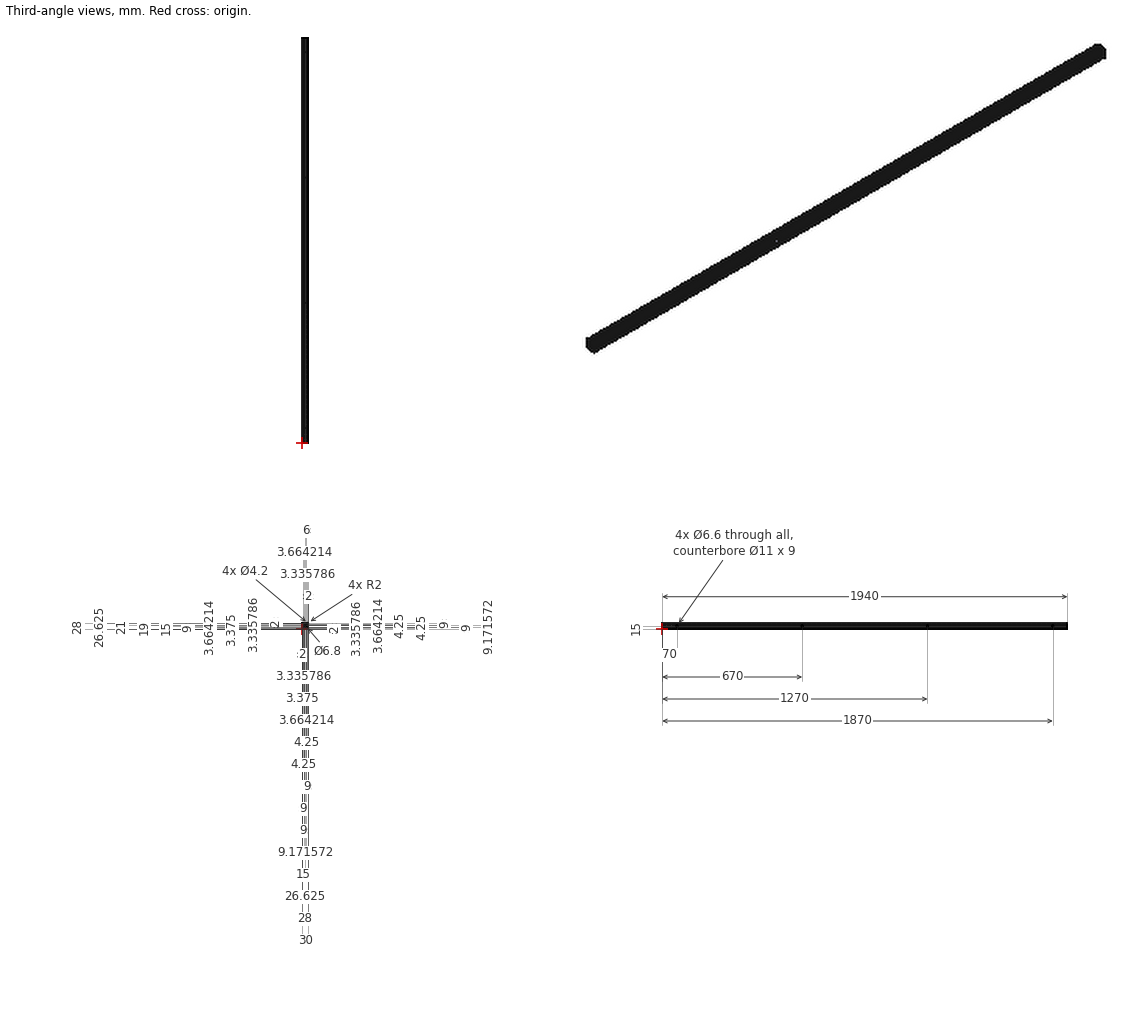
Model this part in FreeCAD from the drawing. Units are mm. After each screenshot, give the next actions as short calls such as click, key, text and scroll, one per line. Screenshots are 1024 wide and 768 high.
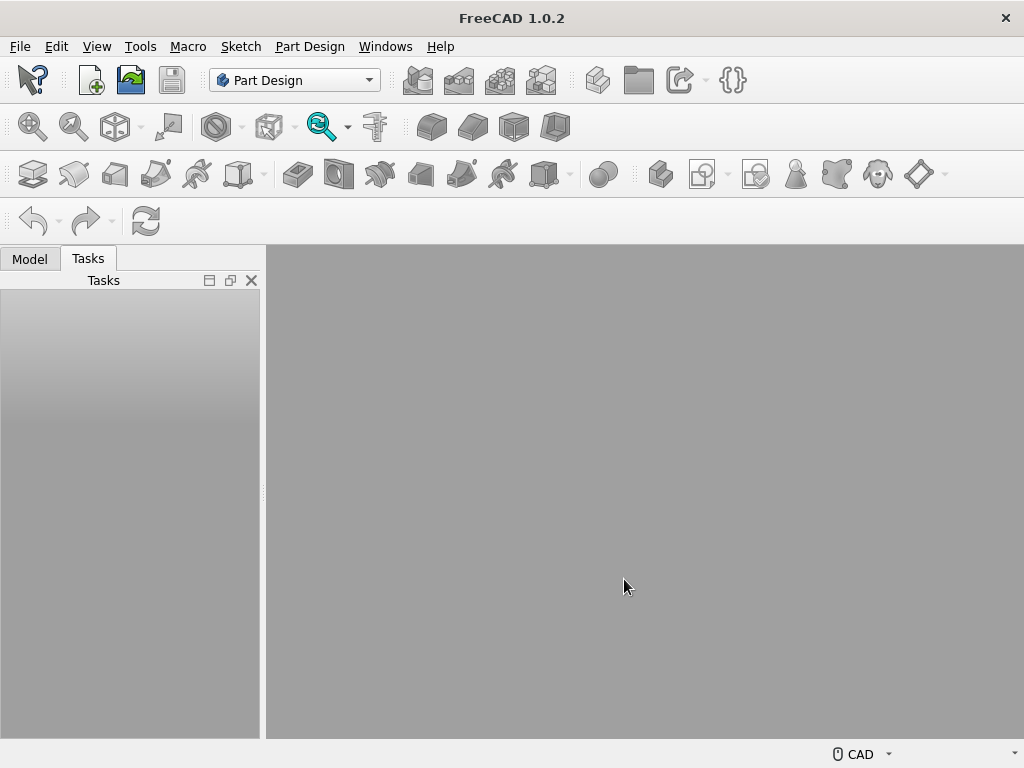
key(ctrl+n)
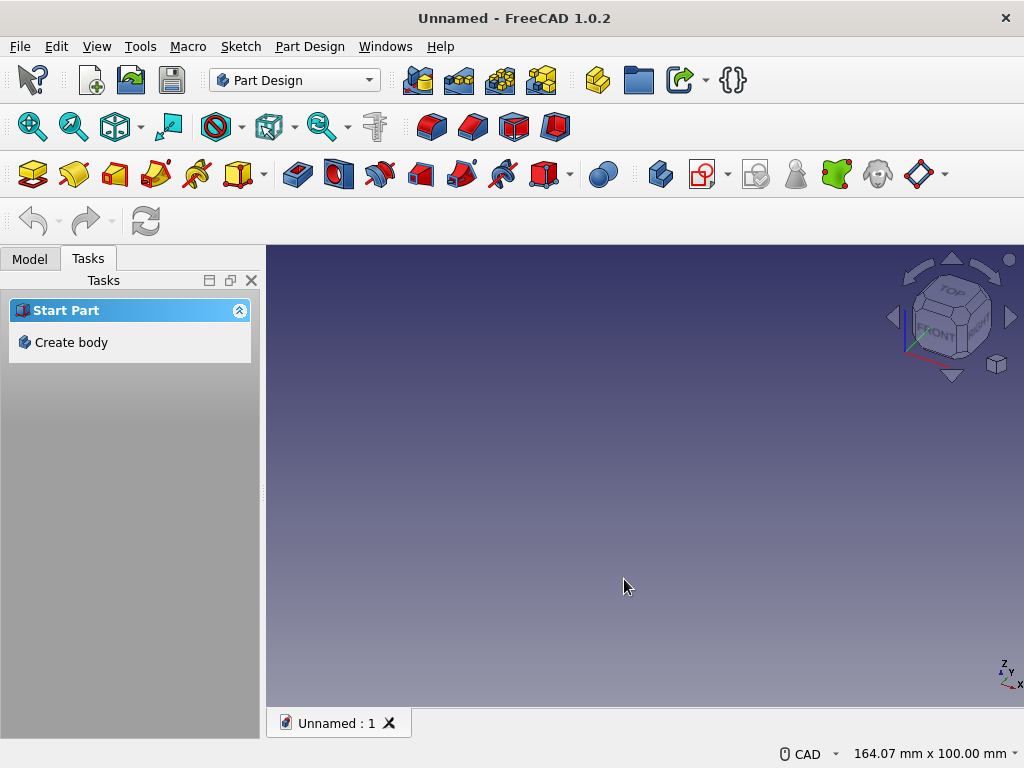
click(702, 174)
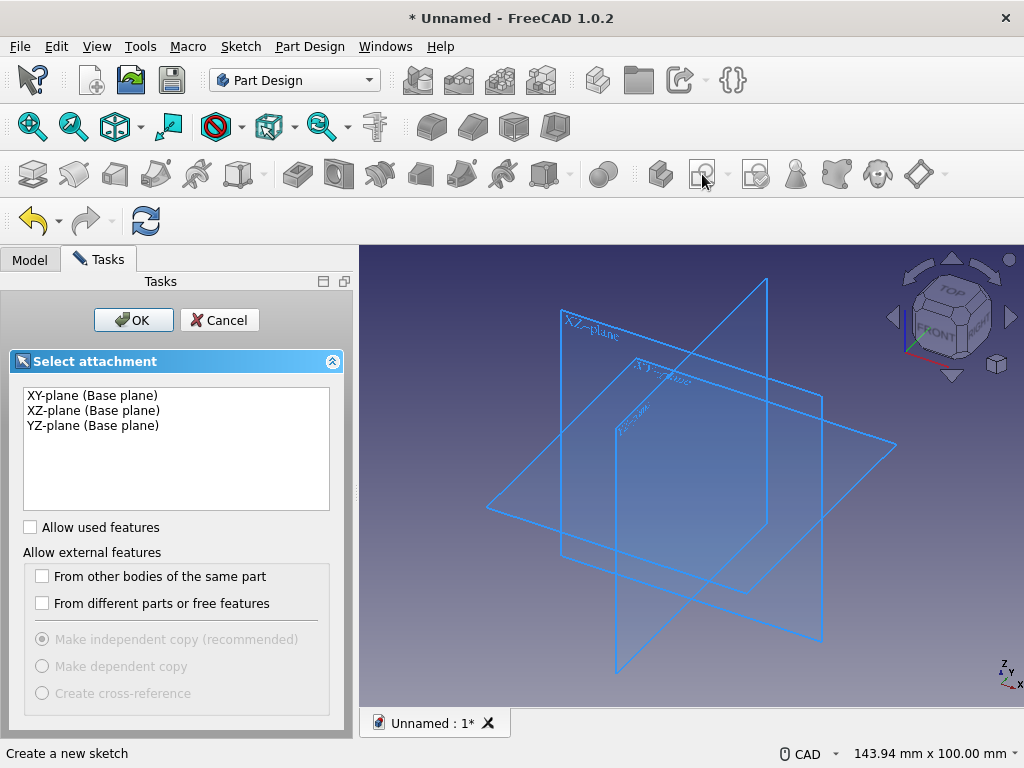
click(84, 410)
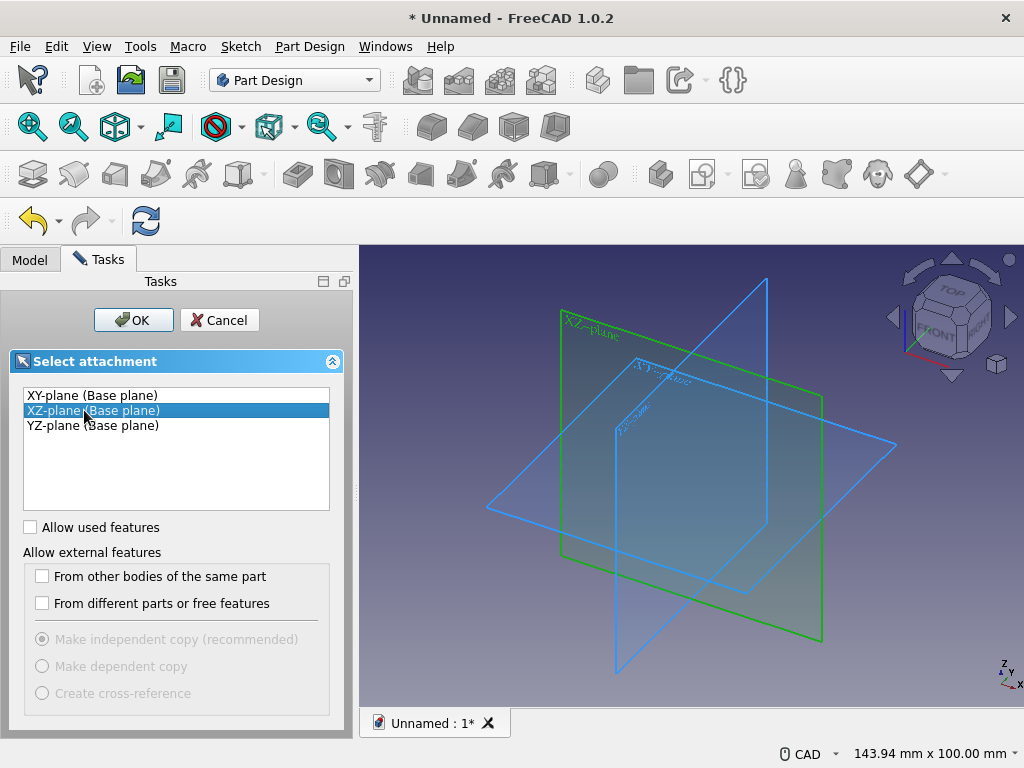
click(134, 320)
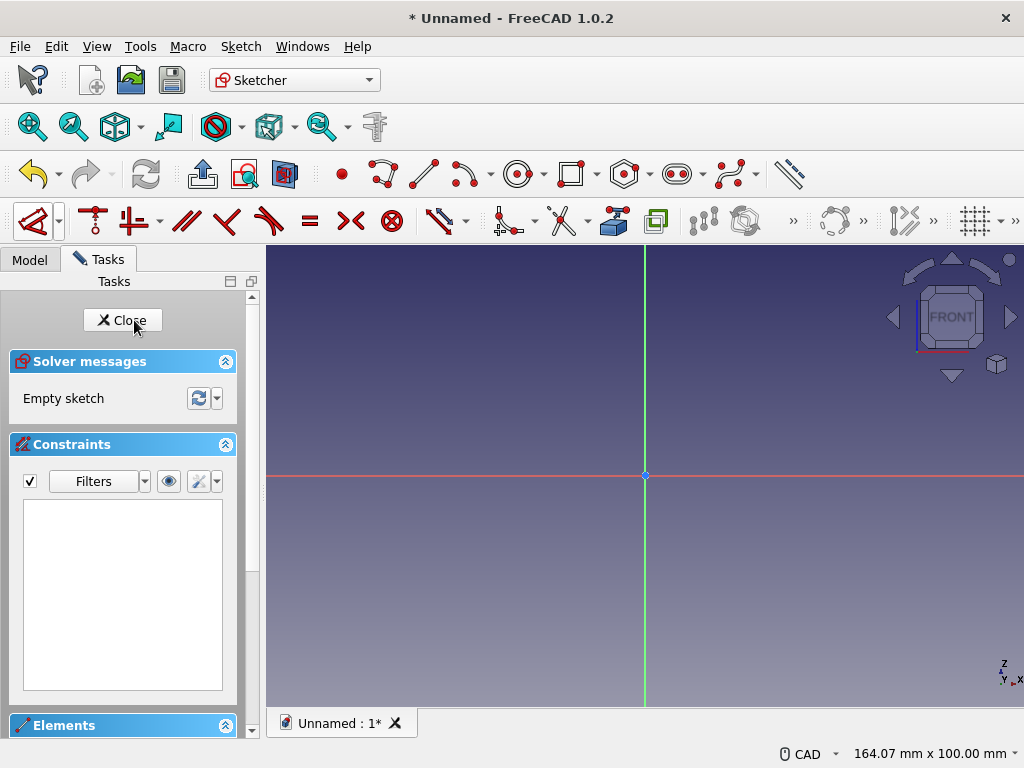
scroll(827, 350, up, 4)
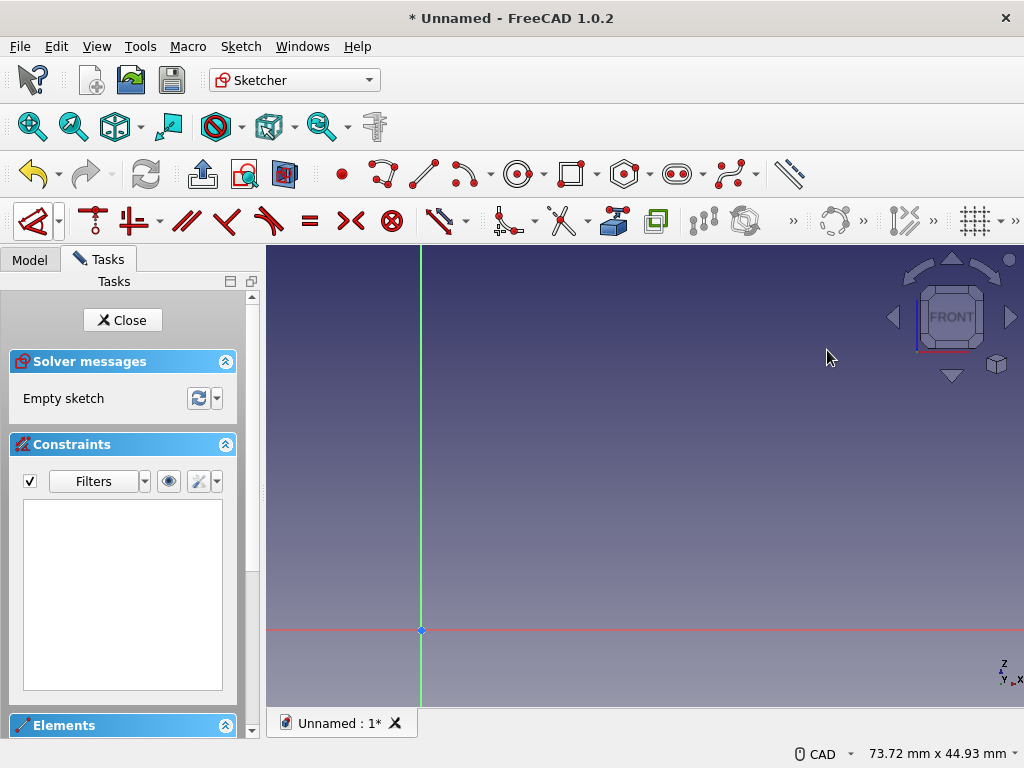
key(g)
key(m)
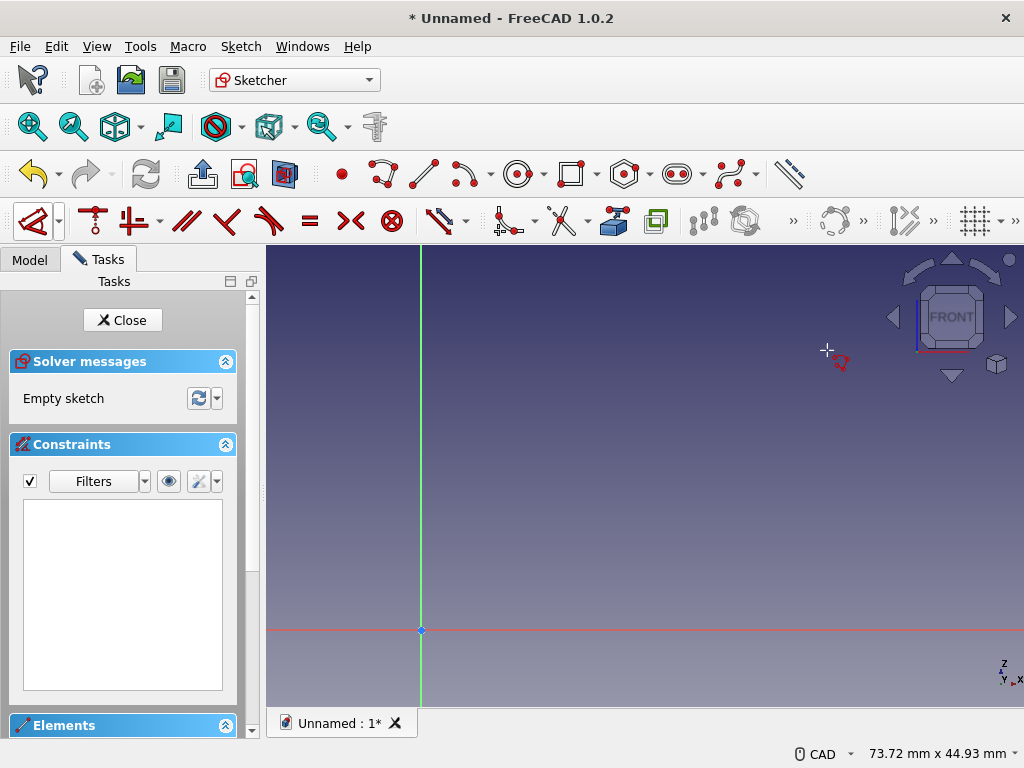
click(730, 342)
click(730, 435)
click(709, 435)
click(709, 391)
click(675, 391)
click(637, 429)
click(637, 523)
click(675, 561)
click(709, 561)
click(709, 517)
click(730, 517)
click(730, 610)
right_click(730, 610)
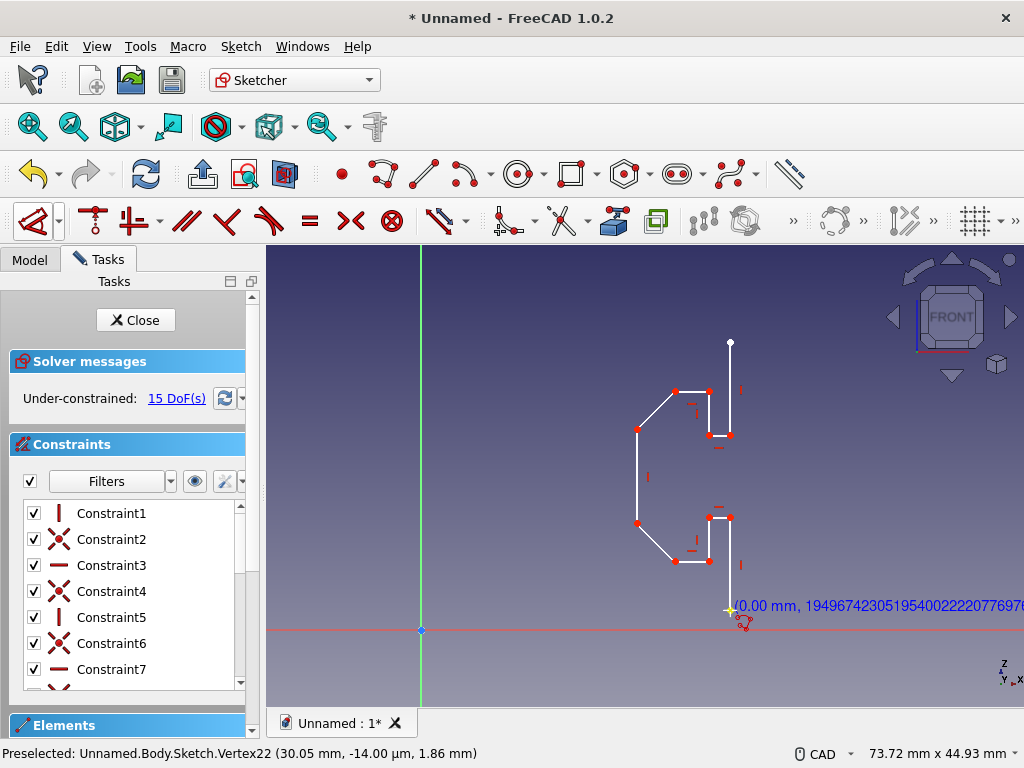
click(709, 630)
click(616, 621)
click(616, 610)
click(660, 610)
click(660, 575)
click(622, 538)
click(528, 538)
click(490, 575)
click(490, 610)
click(534, 610)
click(534, 630)
click(442, 621)
right_click(442, 621)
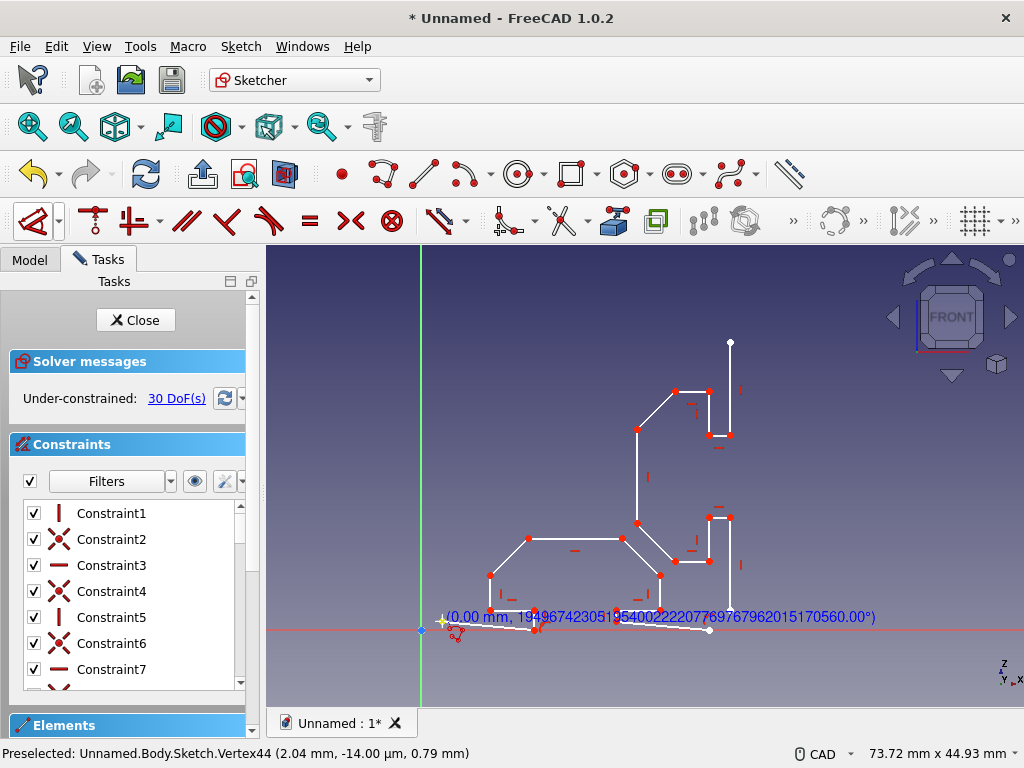
click(421, 610)
click(430, 517)
click(442, 517)
click(442, 561)
click(476, 561)
click(514, 523)
click(514, 429)
click(476, 391)
click(442, 391)
click(442, 435)
click(421, 435)
click(430, 342)
right_click(430, 342)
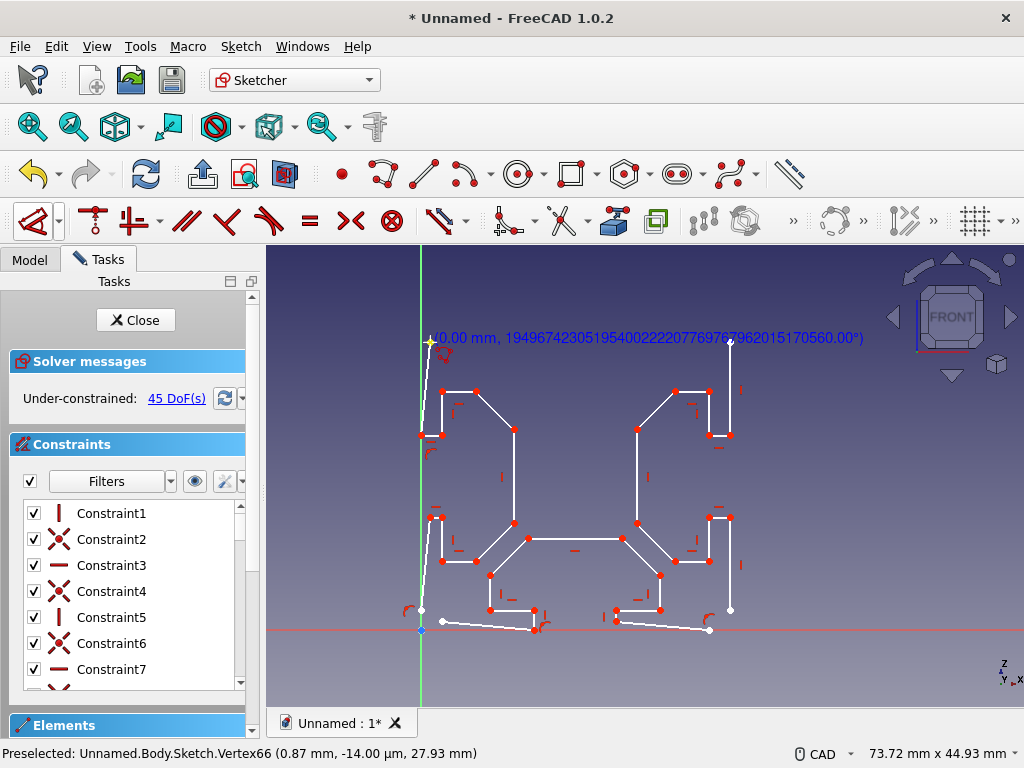
click(442, 322)
click(534, 322)
click(534, 342)
click(490, 342)
click(490, 377)
click(528, 414)
click(622, 414)
click(660, 377)
click(660, 342)
click(616, 342)
click(616, 322)
click(709, 322)
right_click(709, 322)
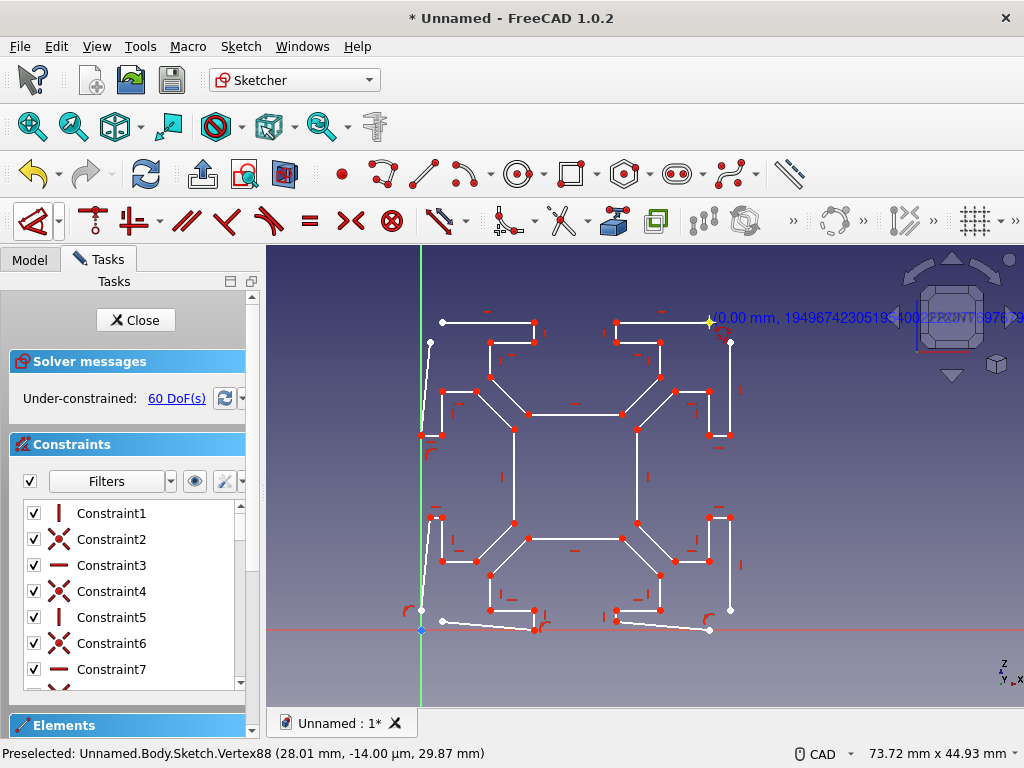
click(490, 174)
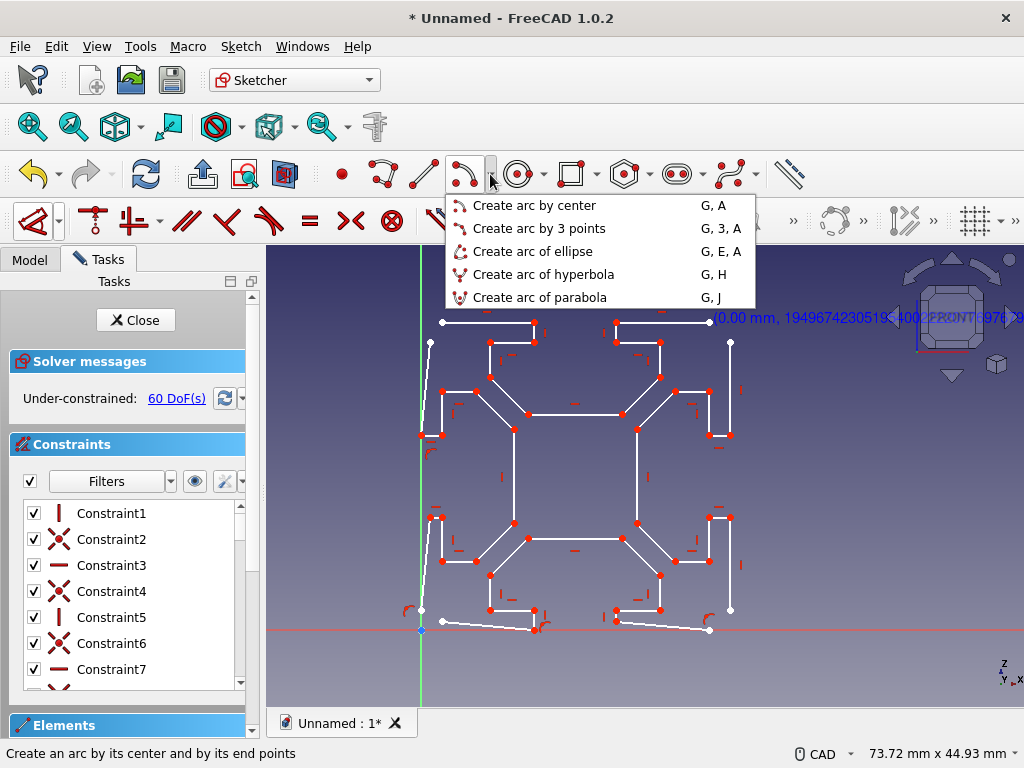
click(600, 228)